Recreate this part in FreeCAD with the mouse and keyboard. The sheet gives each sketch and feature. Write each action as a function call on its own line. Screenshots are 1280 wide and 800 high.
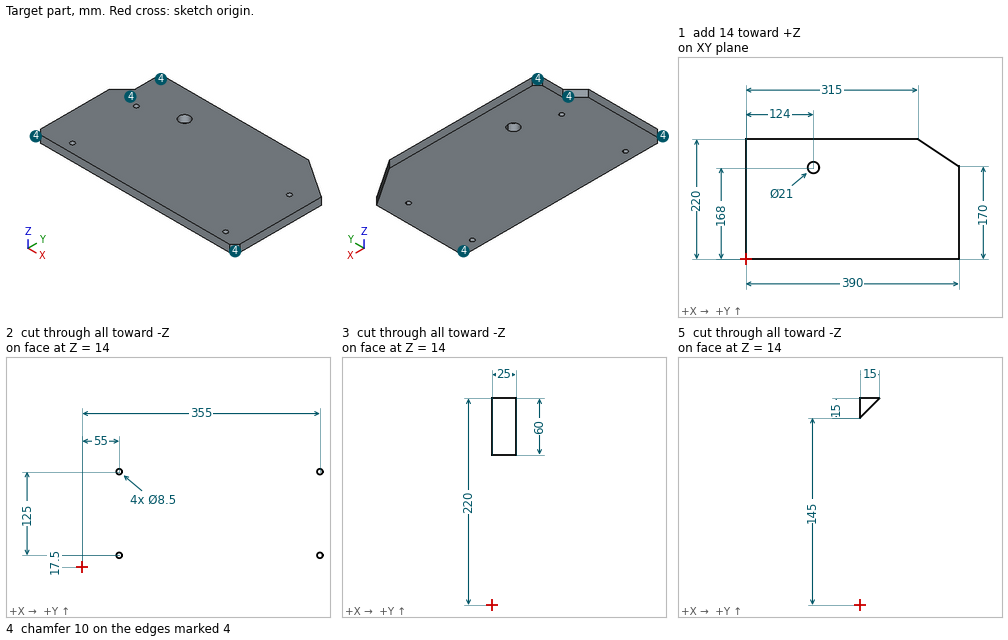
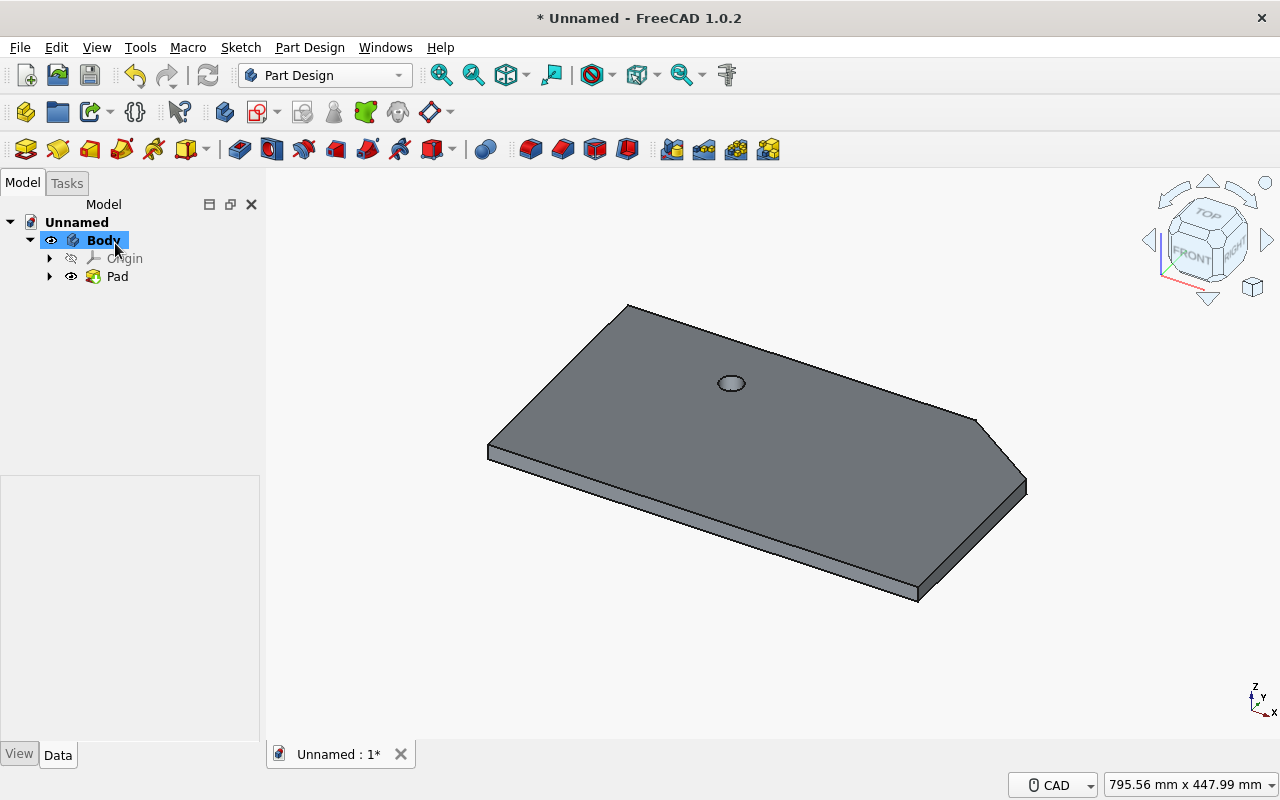
click(834, 466)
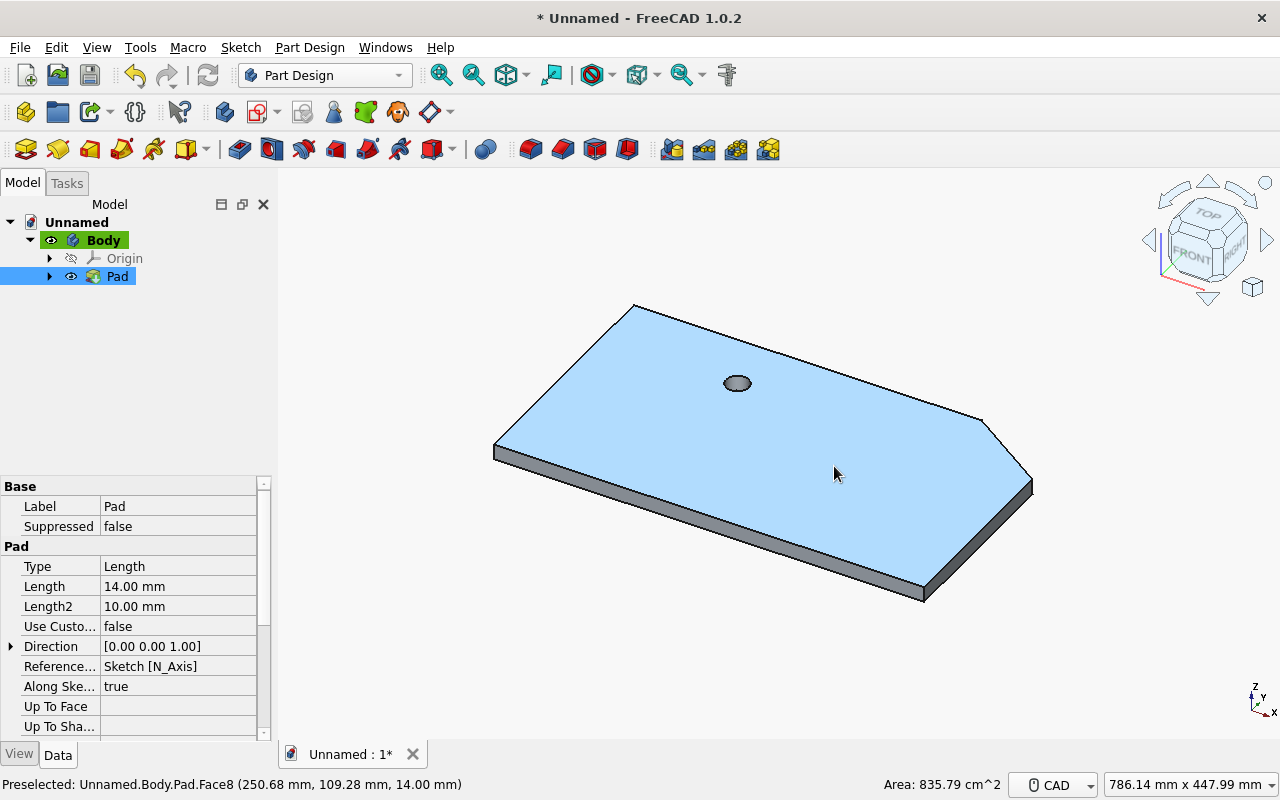
click(258, 112)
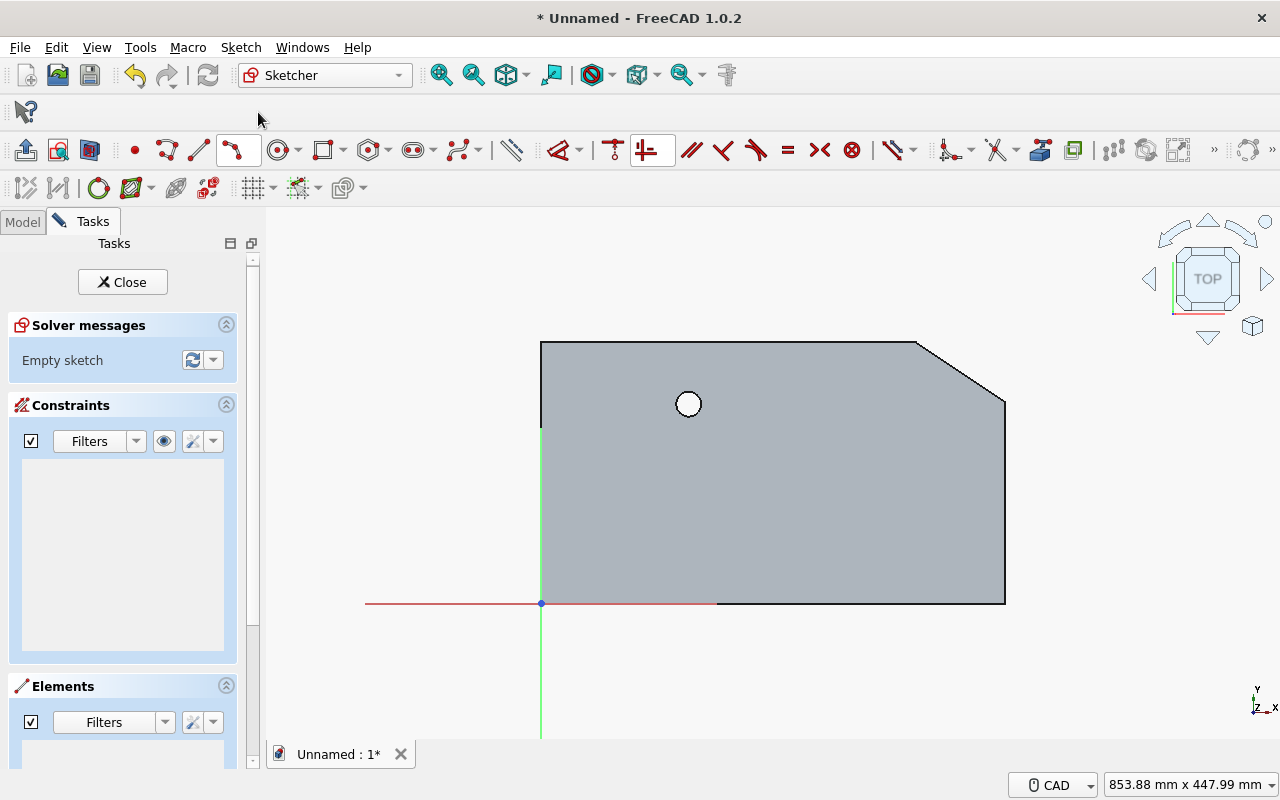
scroll(857, 605, up, 2)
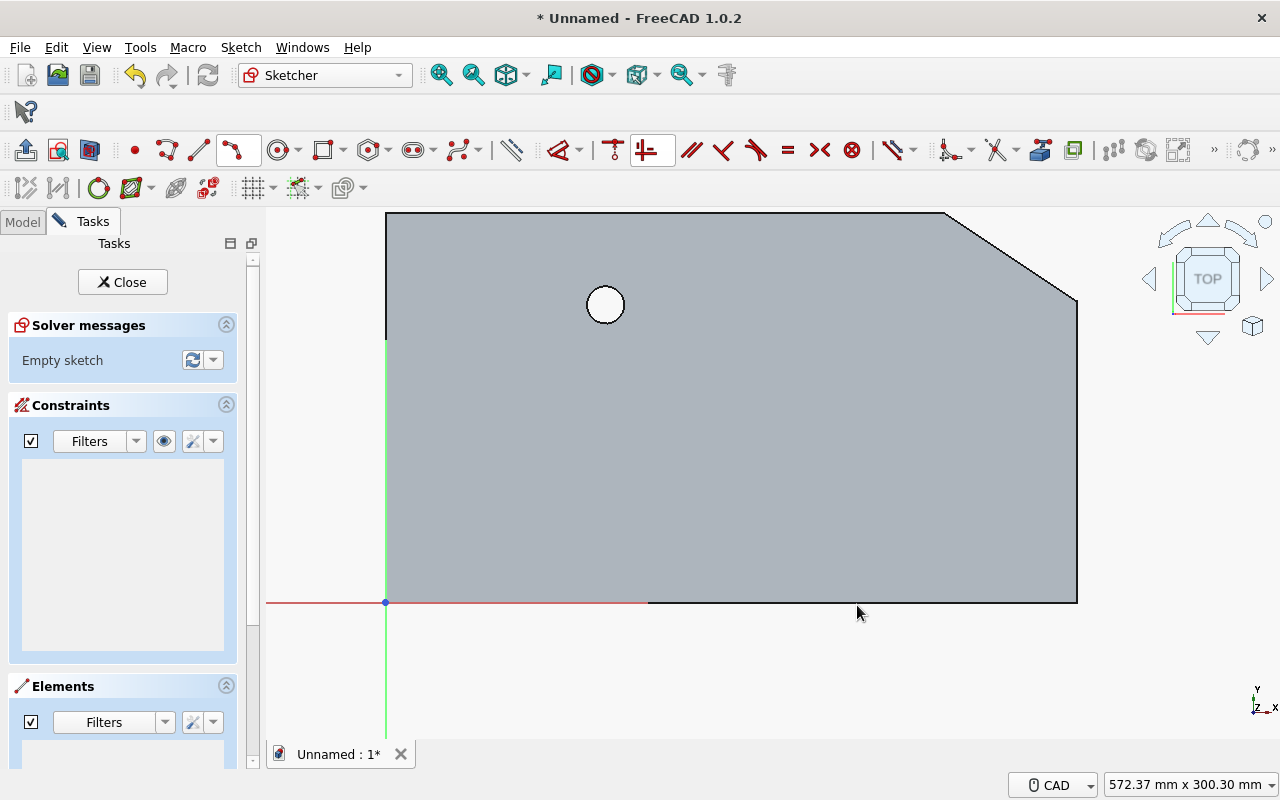
click(278, 150)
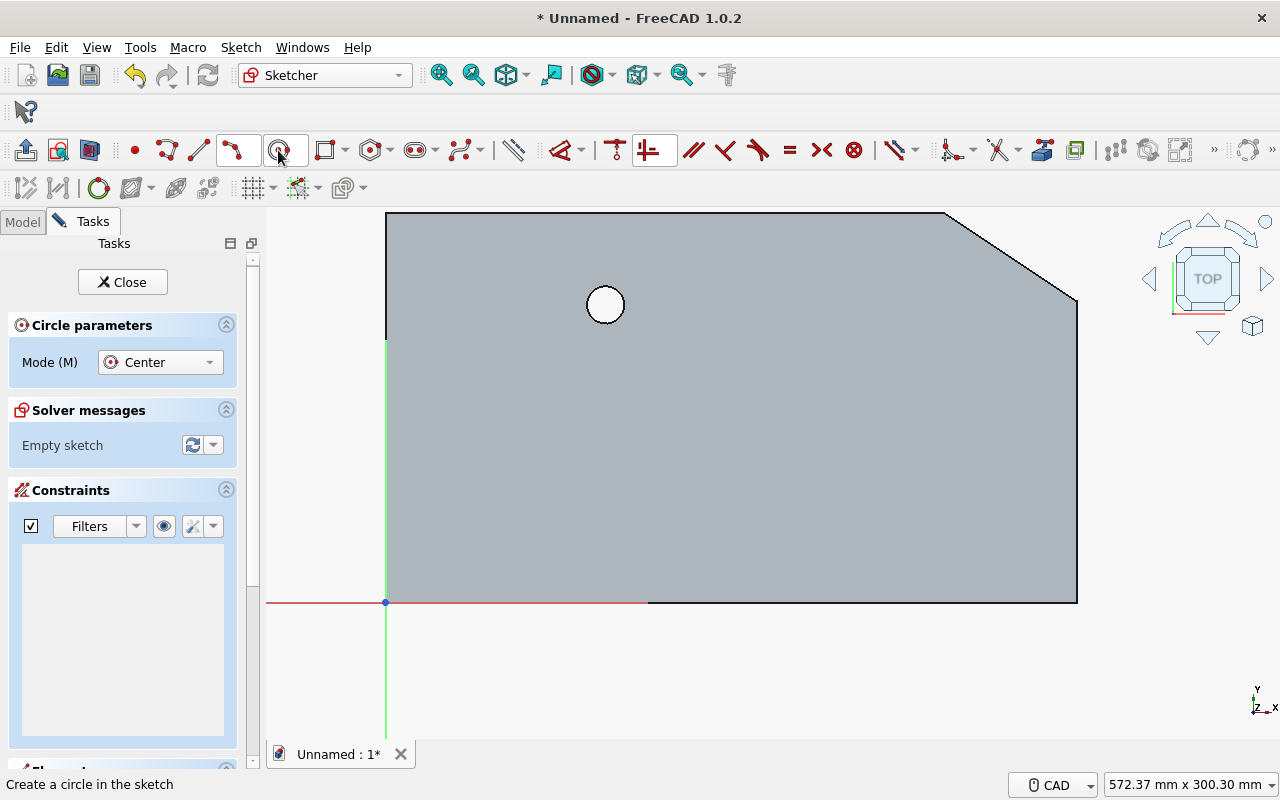
scroll(483, 350, up, 6)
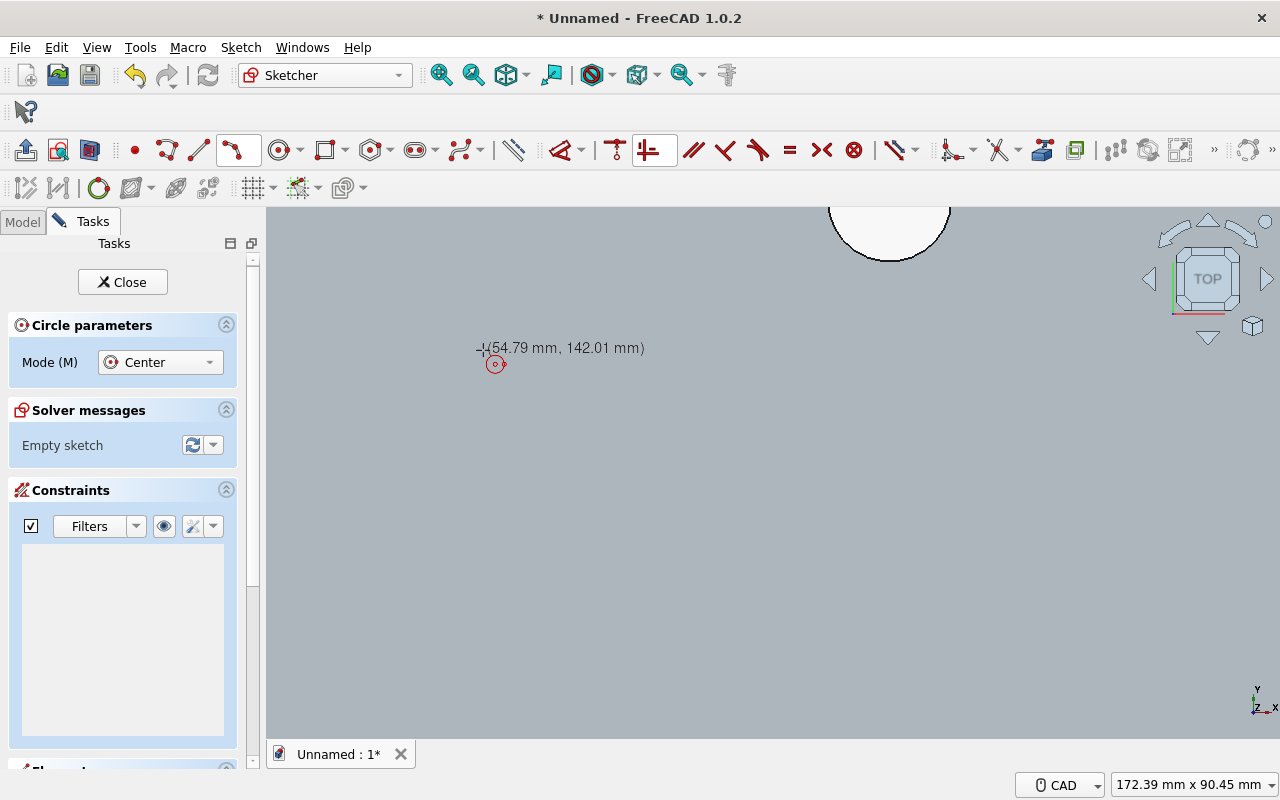
click(484, 350)
move(501, 332)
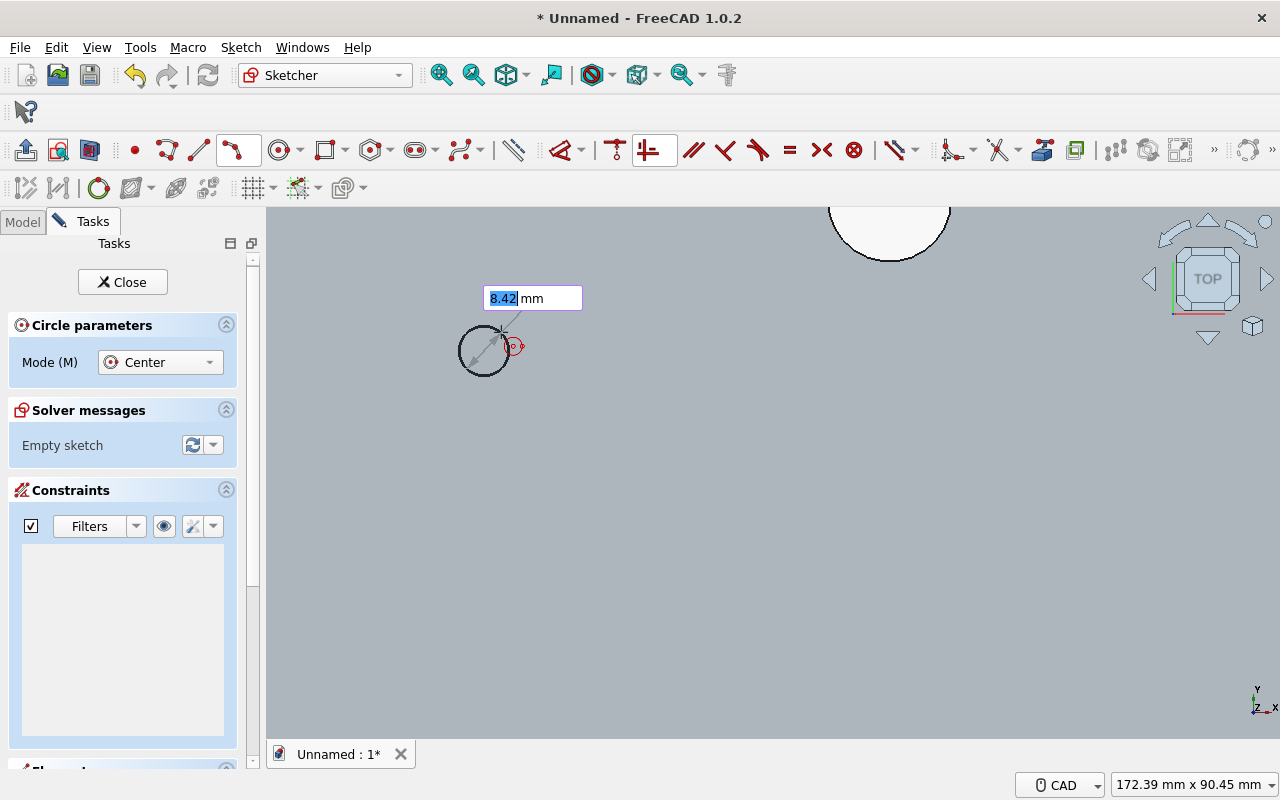
text(8.5)
key(Return)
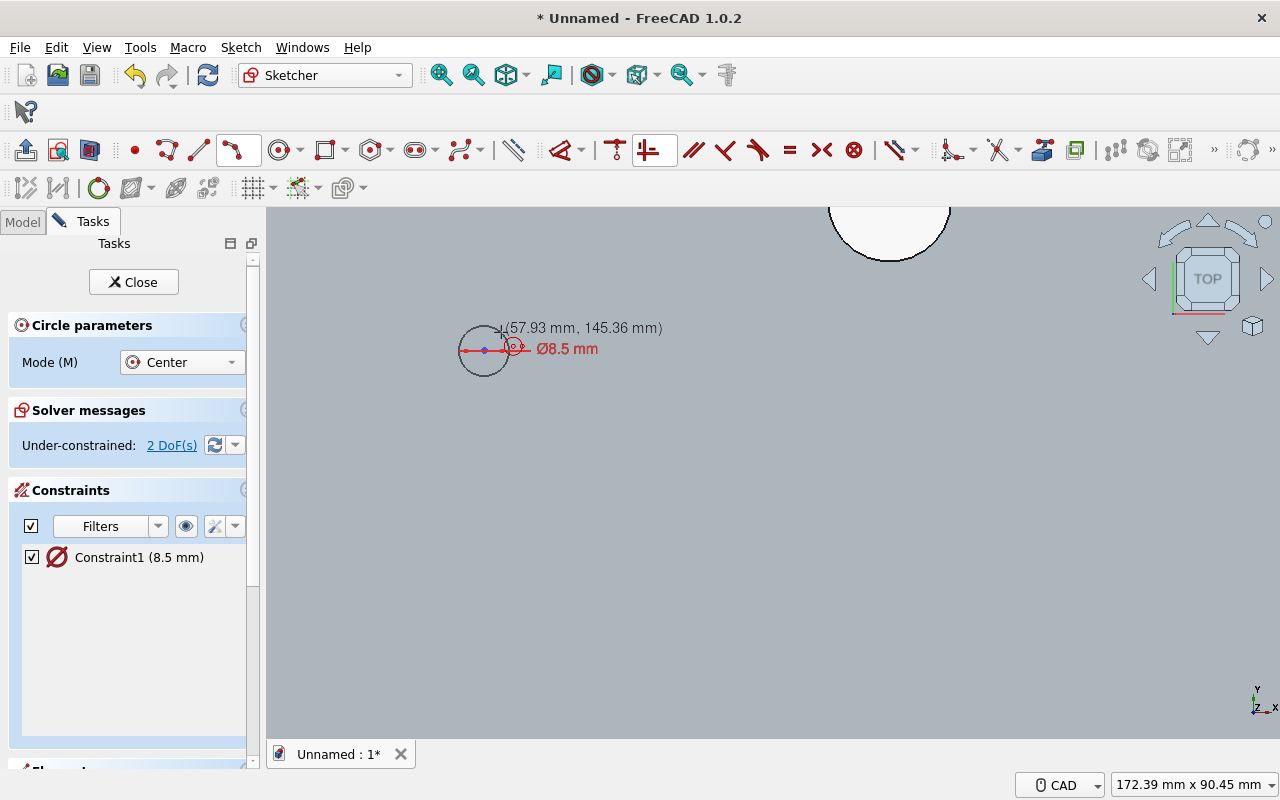
scroll(484, 351, down, 6)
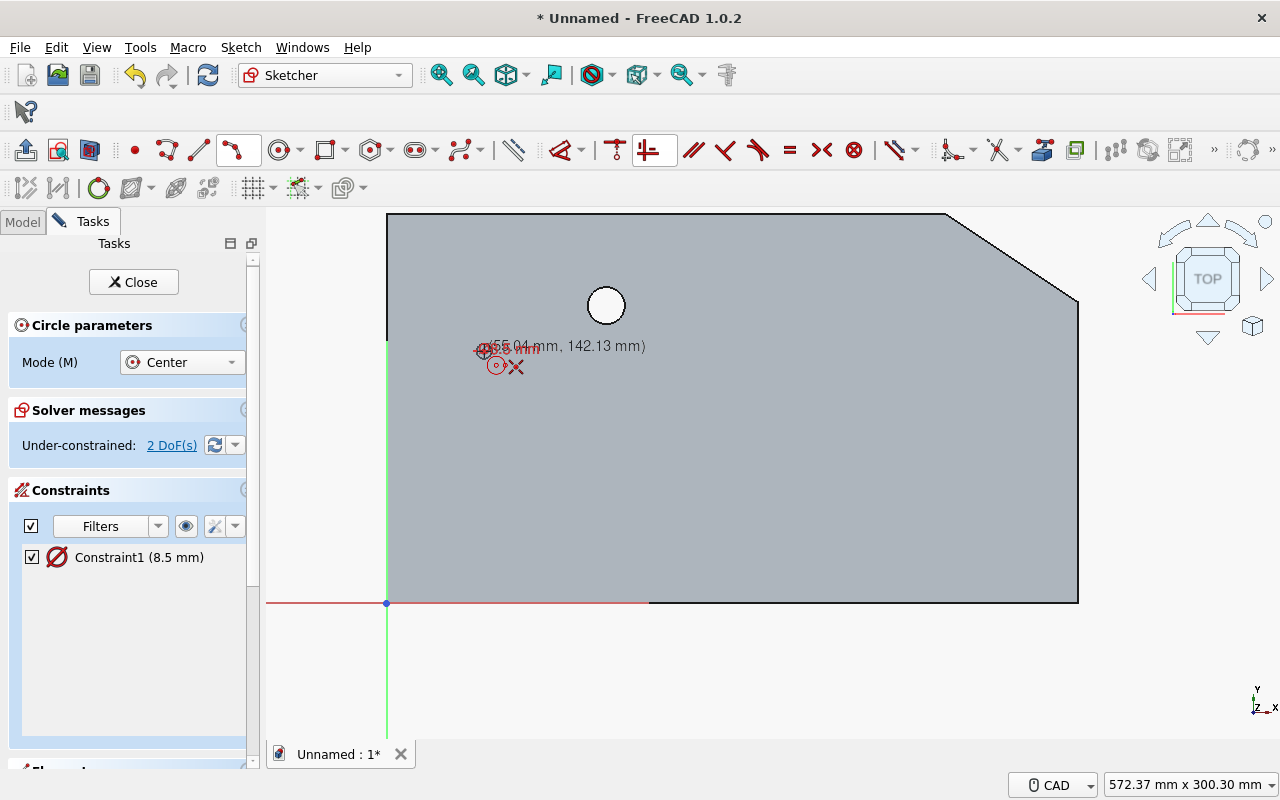
scroll(484, 572, up, 6)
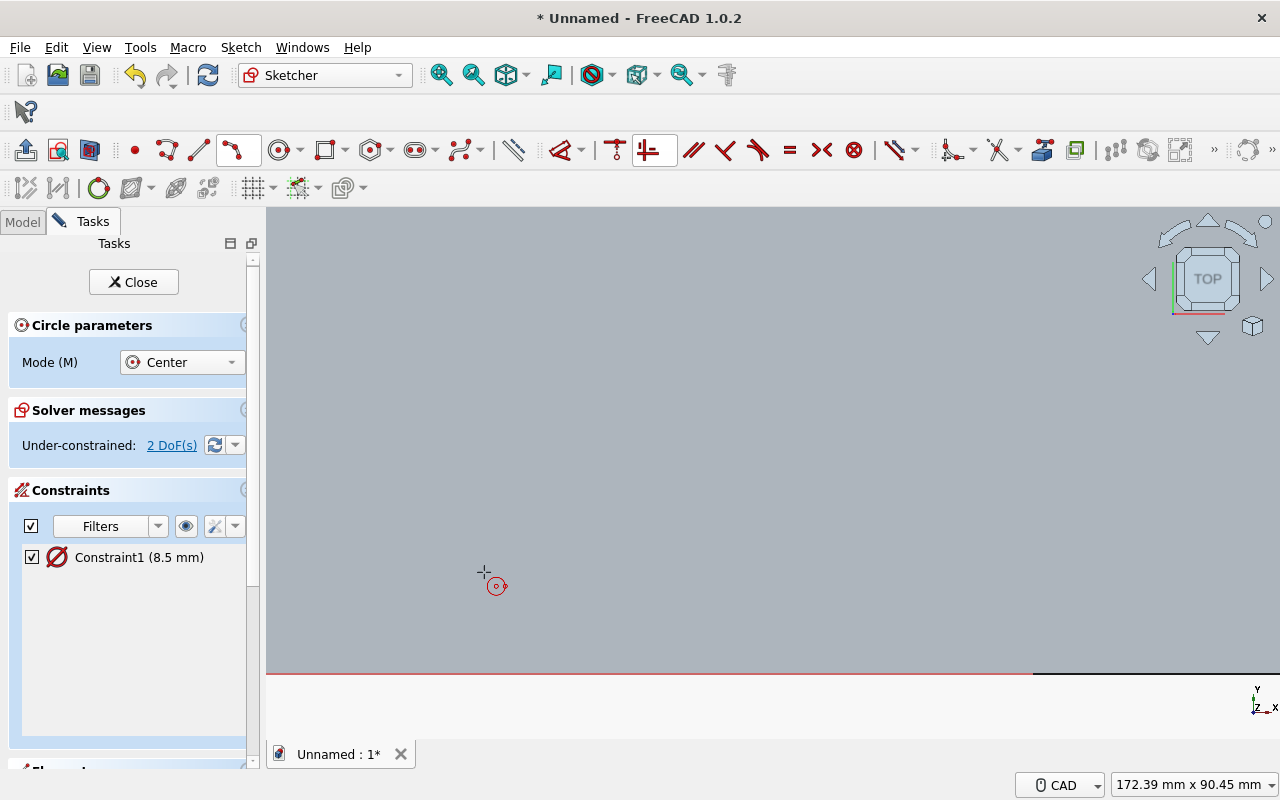
click(484, 571)
move(501, 554)